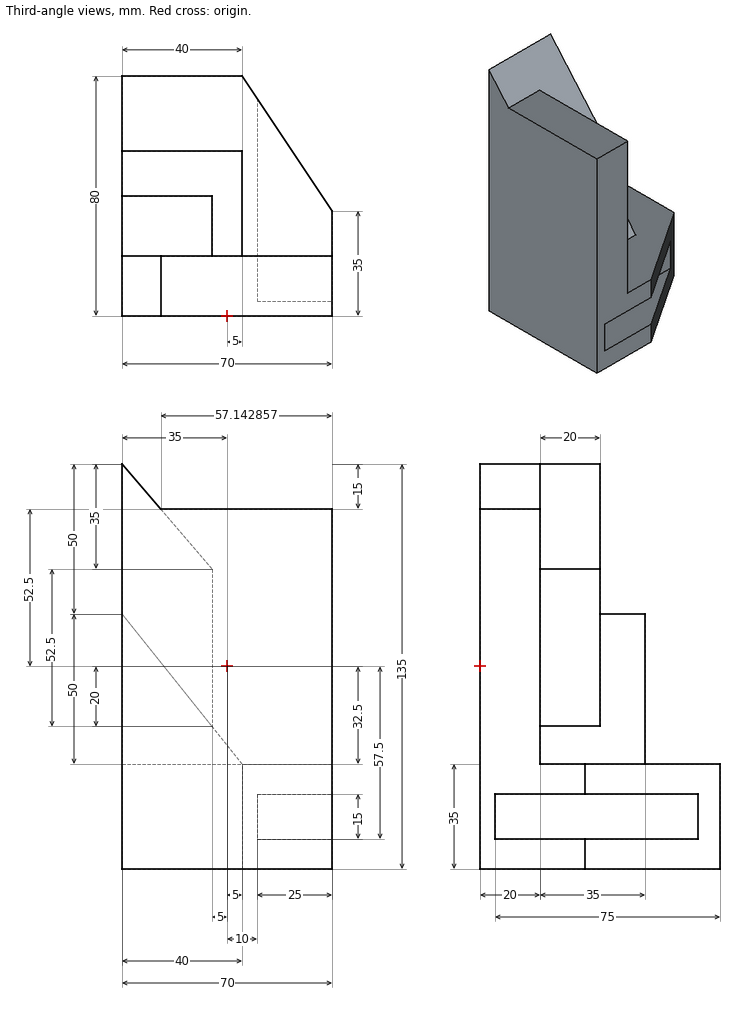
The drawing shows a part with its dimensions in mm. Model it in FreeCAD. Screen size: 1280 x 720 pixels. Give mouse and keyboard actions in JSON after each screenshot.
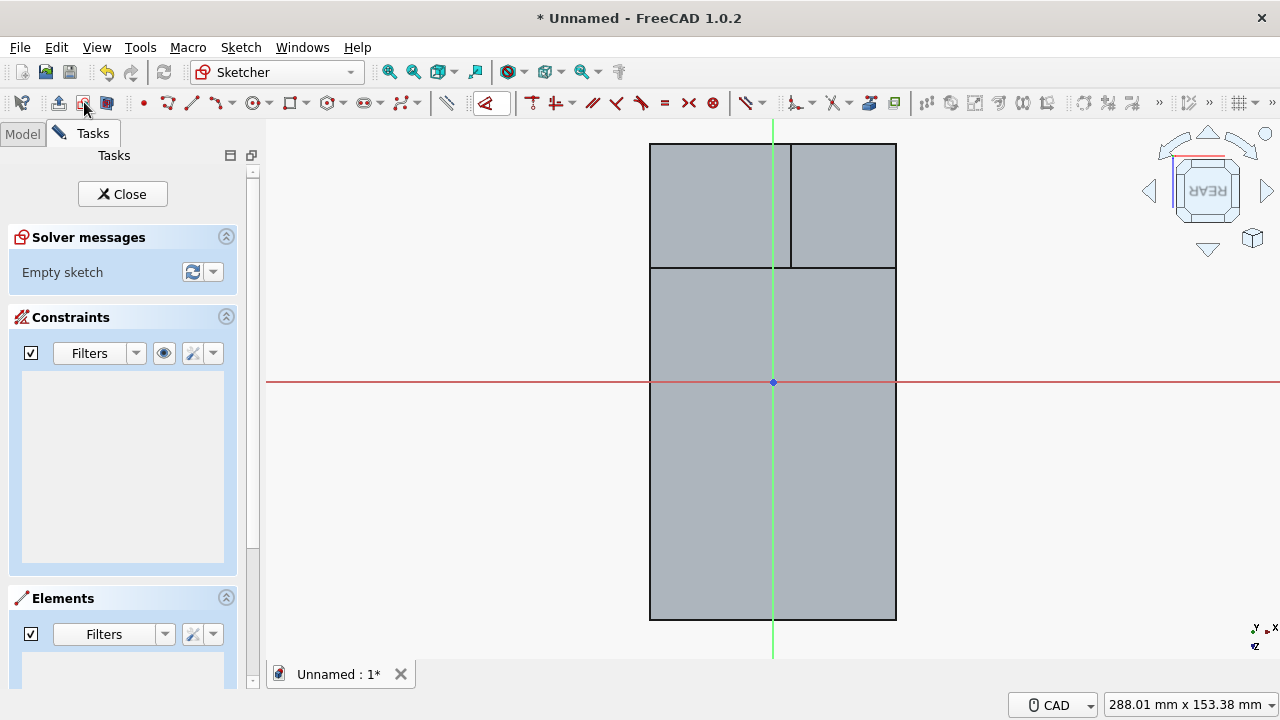
{"action": "scroll", "coordinate": [993, 149], "scroll_direction": "up", "scroll_amount": 3}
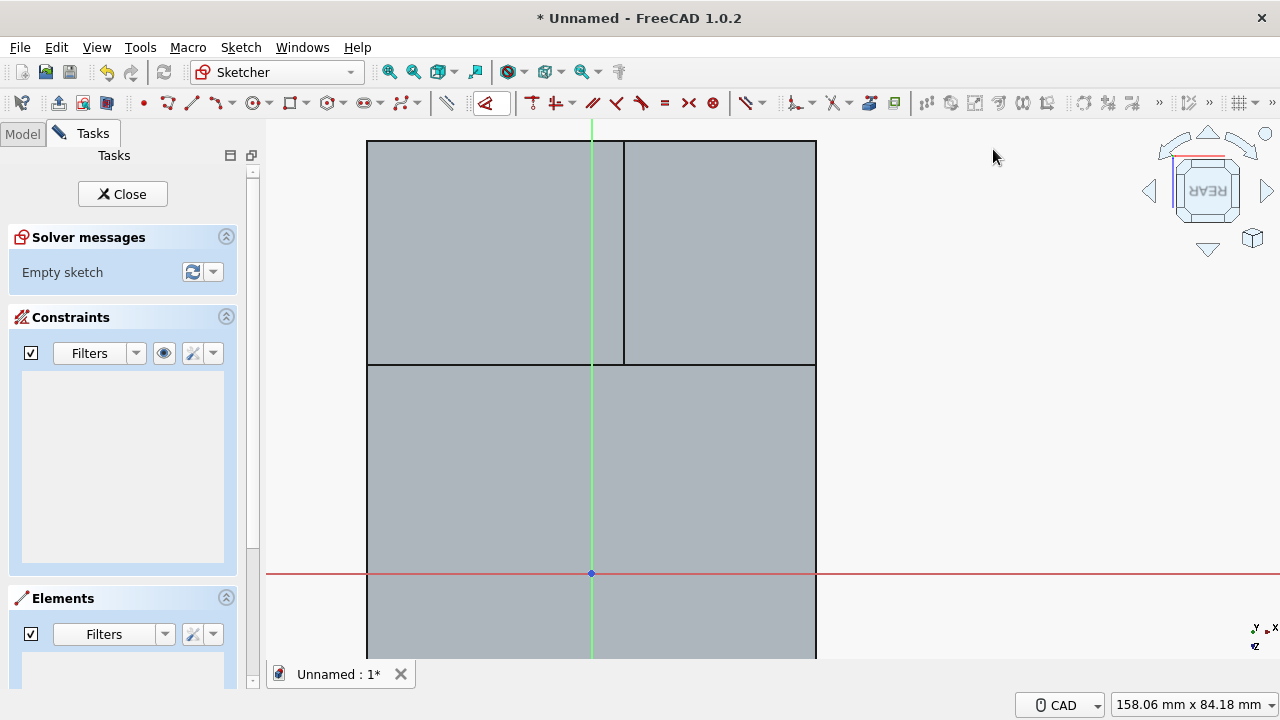
{"action": "left_click", "coordinate": [290, 104]}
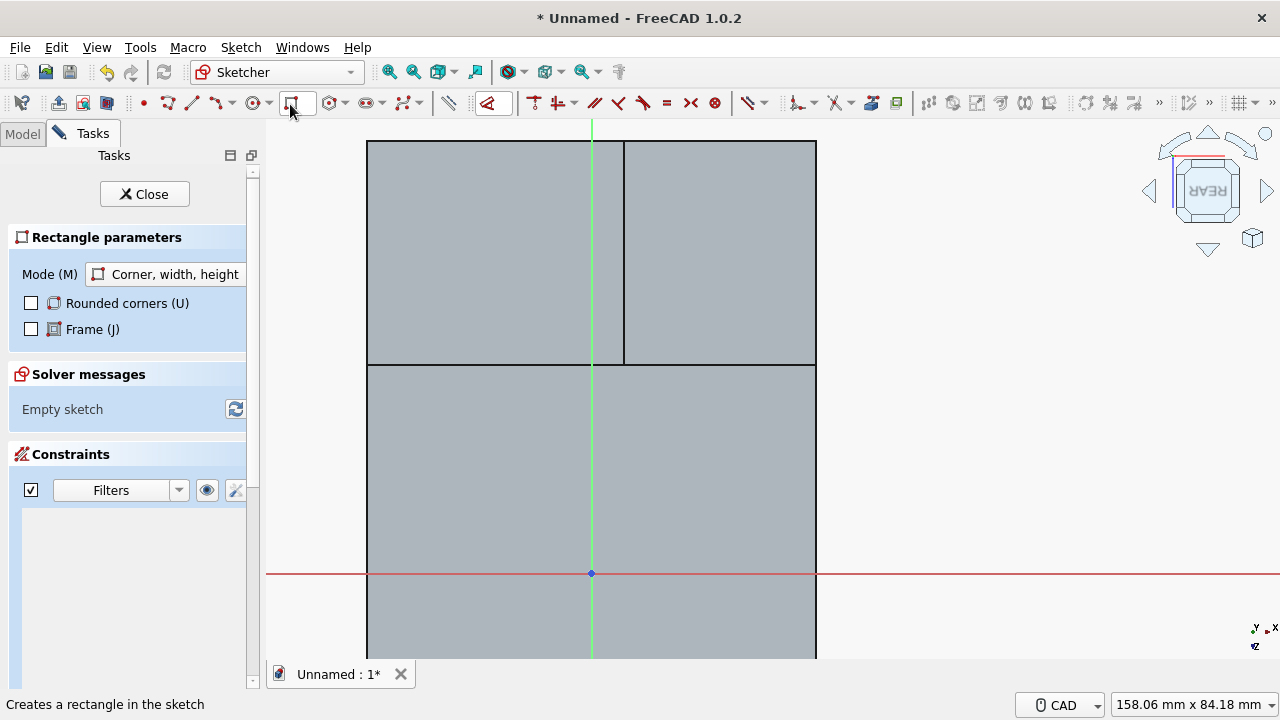
{"action": "left_click", "coordinate": [656, 205]}
{"action": "left_click", "coordinate": [816, 301]}
{"action": "key", "text": "Escape"}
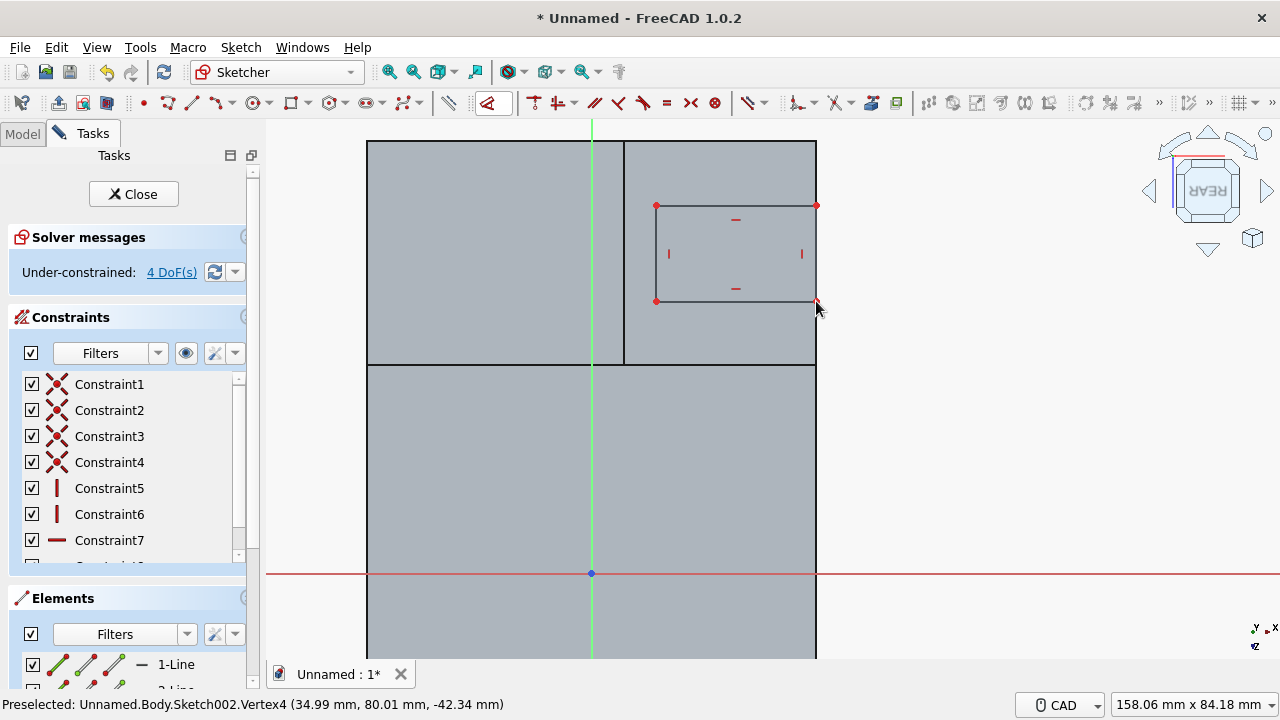
{"action": "left_click", "coordinate": [656, 235]}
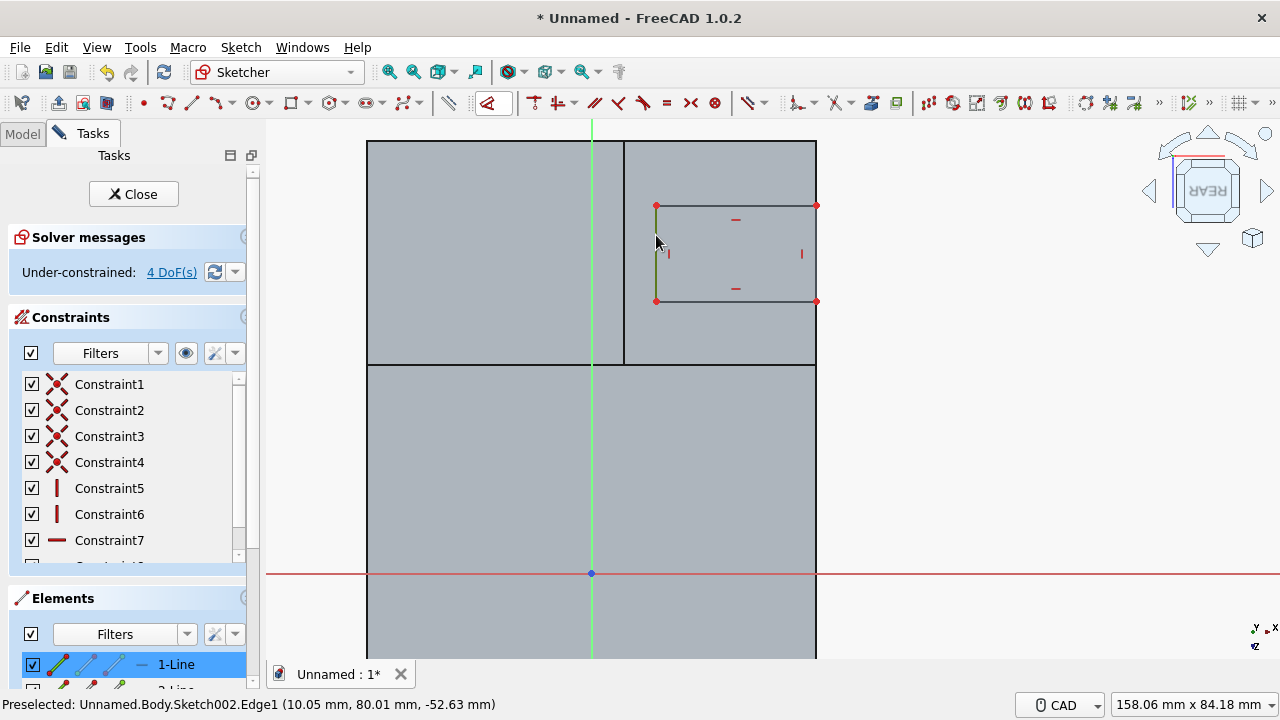
{"action": "left_click", "coordinate": [506, 104]}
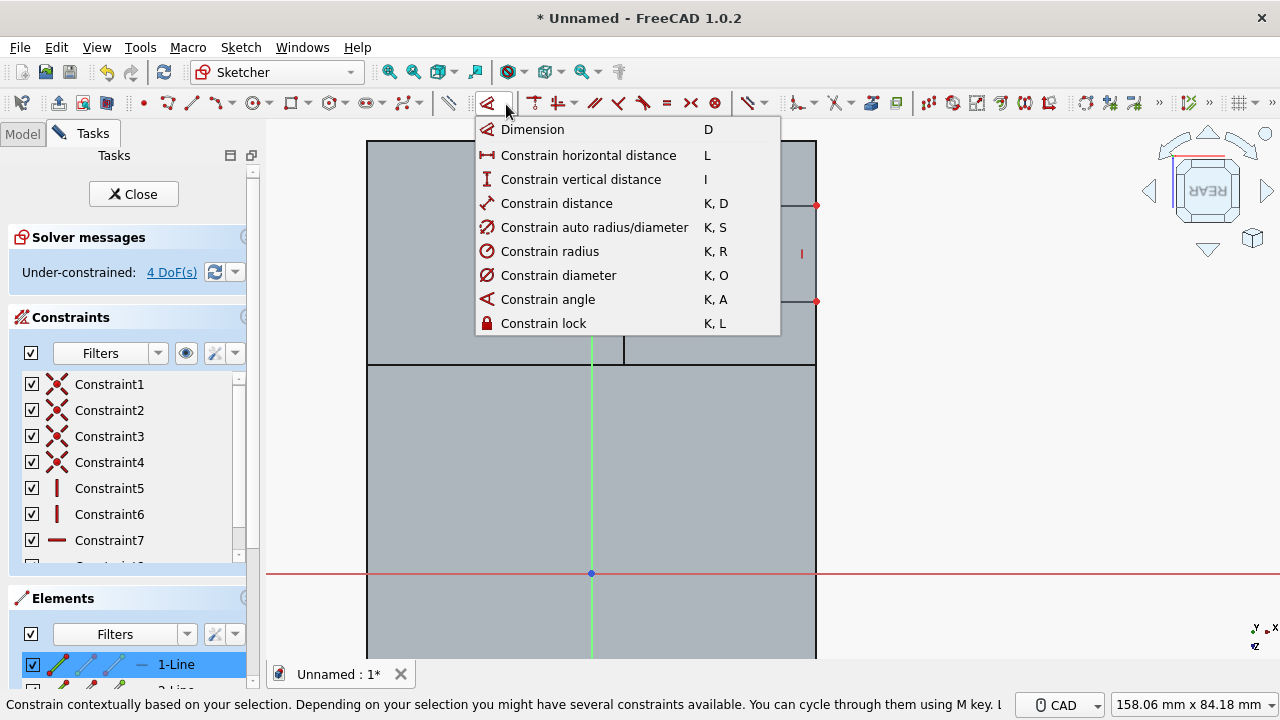
{"action": "left_click", "coordinate": [628, 179]}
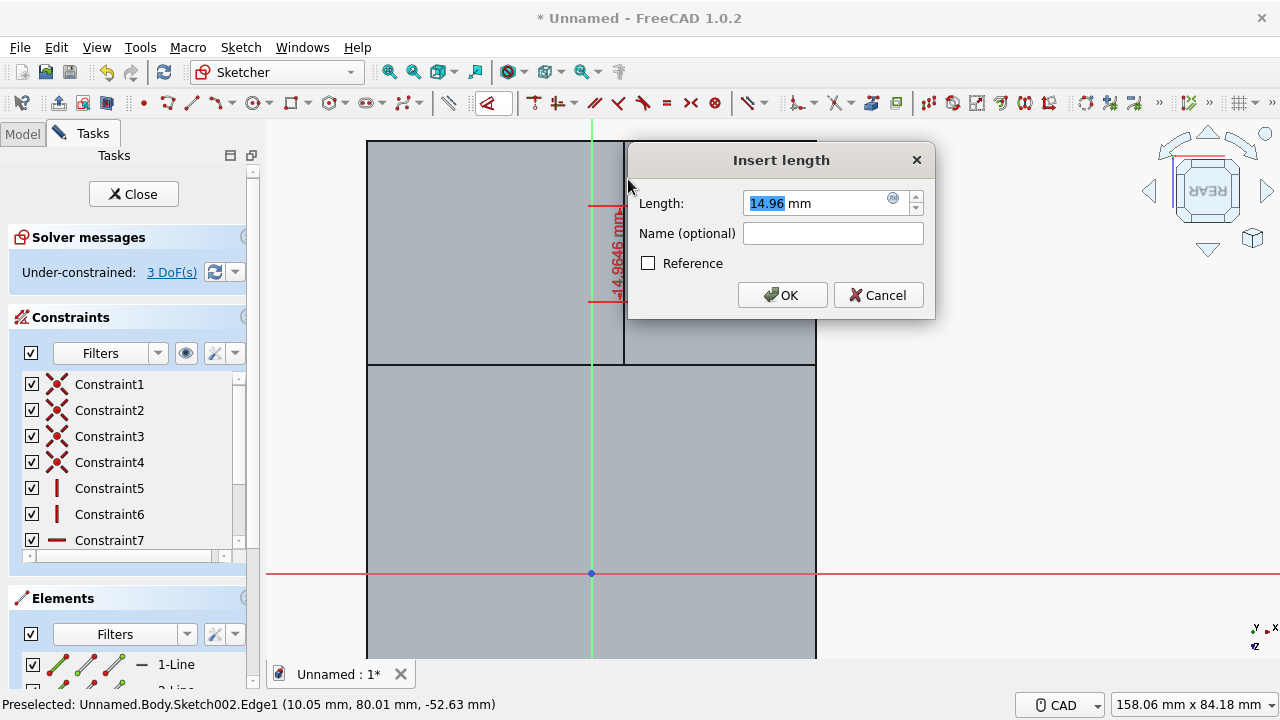
{"action": "type", "text": "15"}
{"action": "key", "text": "Return"}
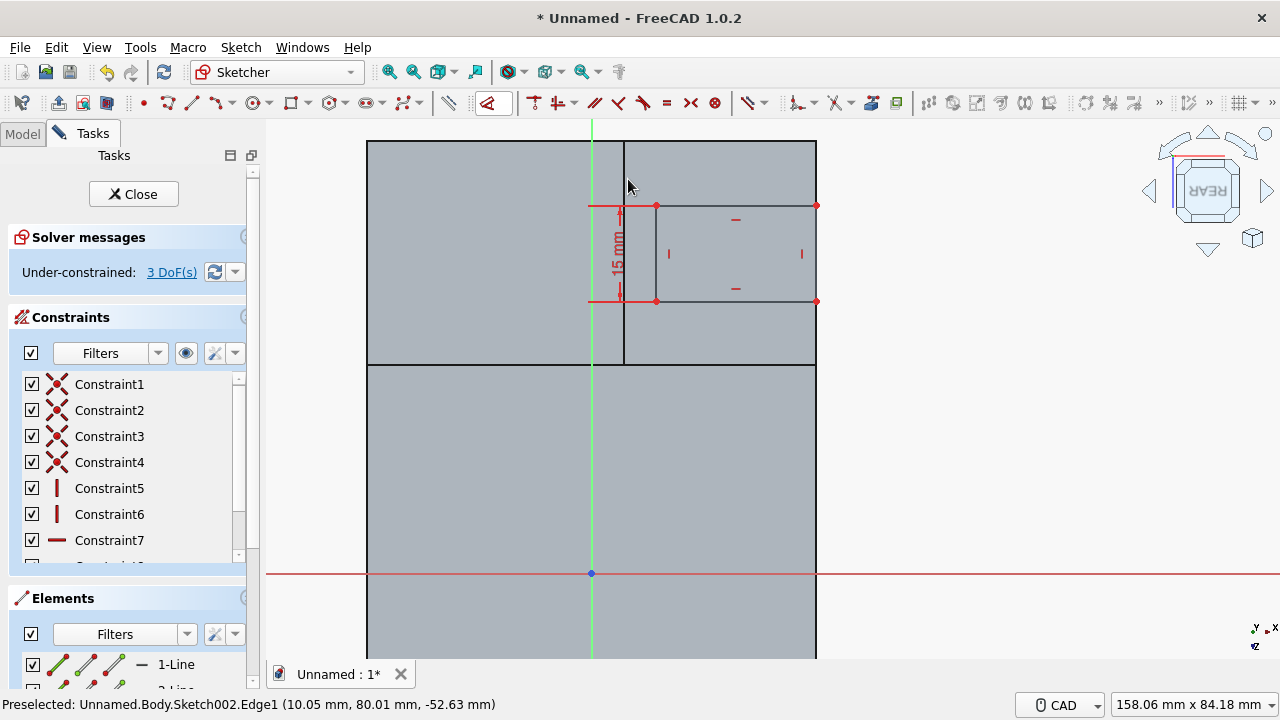
{"action": "left_click", "coordinate": [704, 302]}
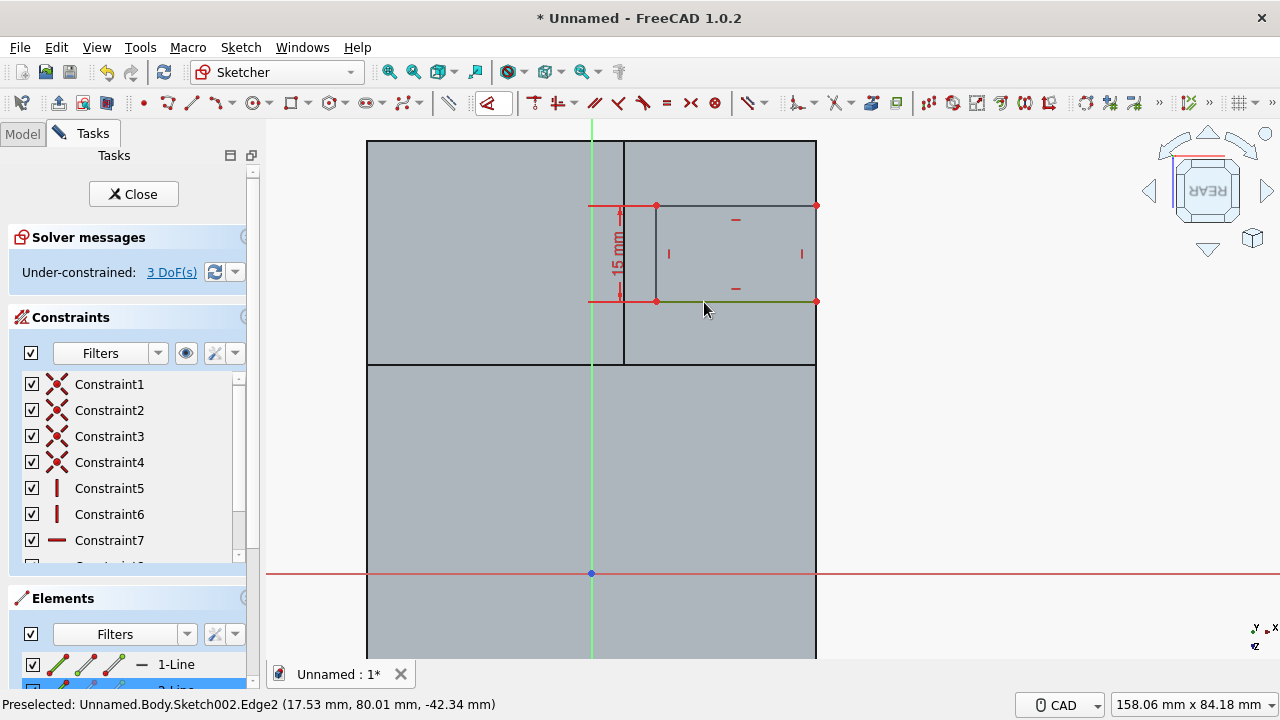
{"action": "left_click", "coordinate": [506, 104]}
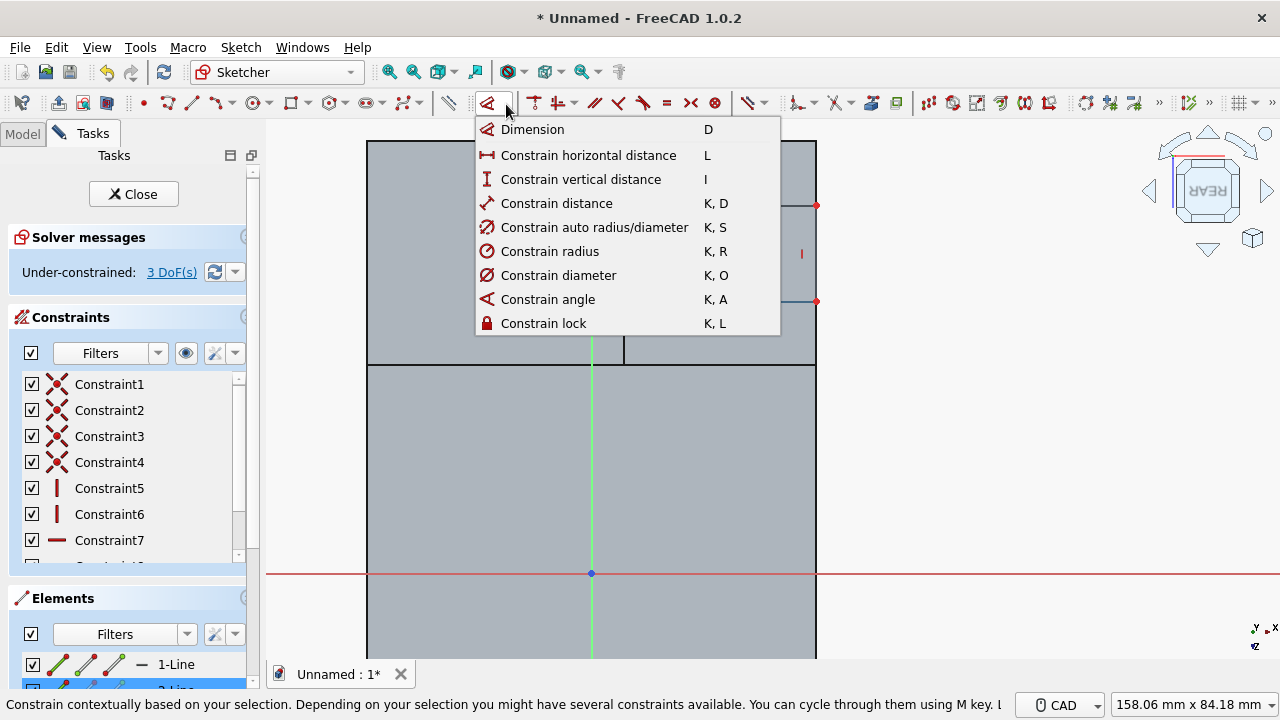
{"action": "left_click", "coordinate": [628, 155]}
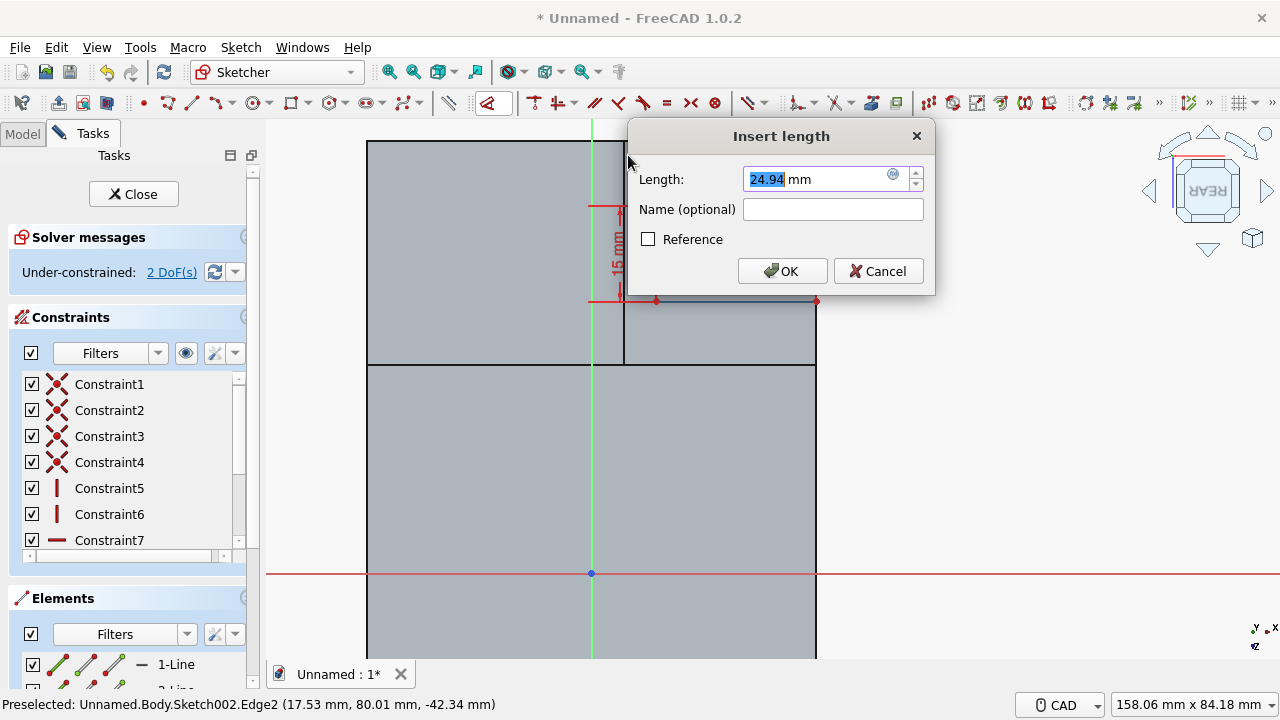
{"action": "type", "text": "25"}
{"action": "key", "text": "Return"}